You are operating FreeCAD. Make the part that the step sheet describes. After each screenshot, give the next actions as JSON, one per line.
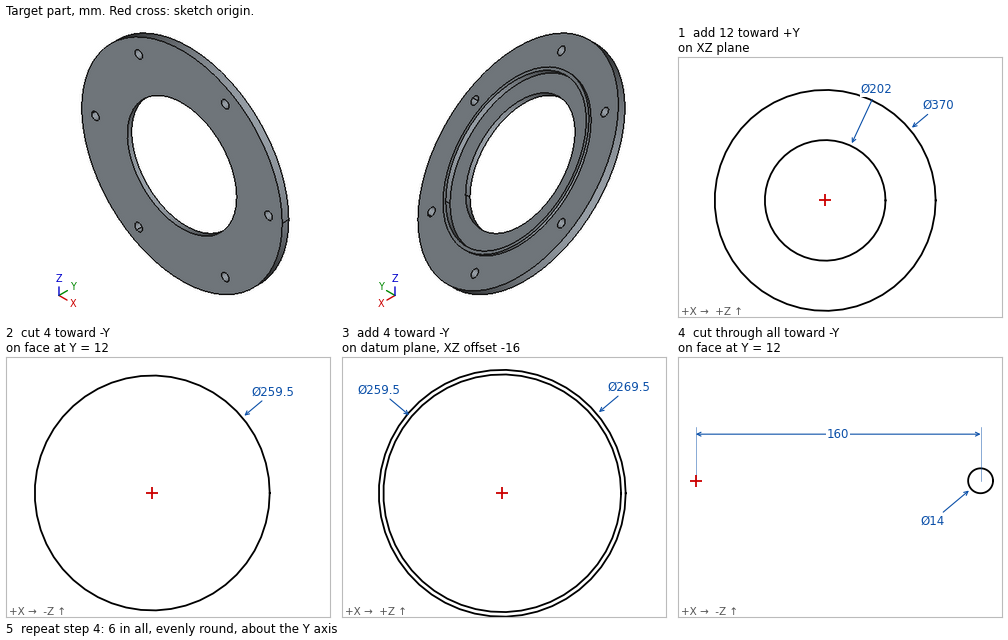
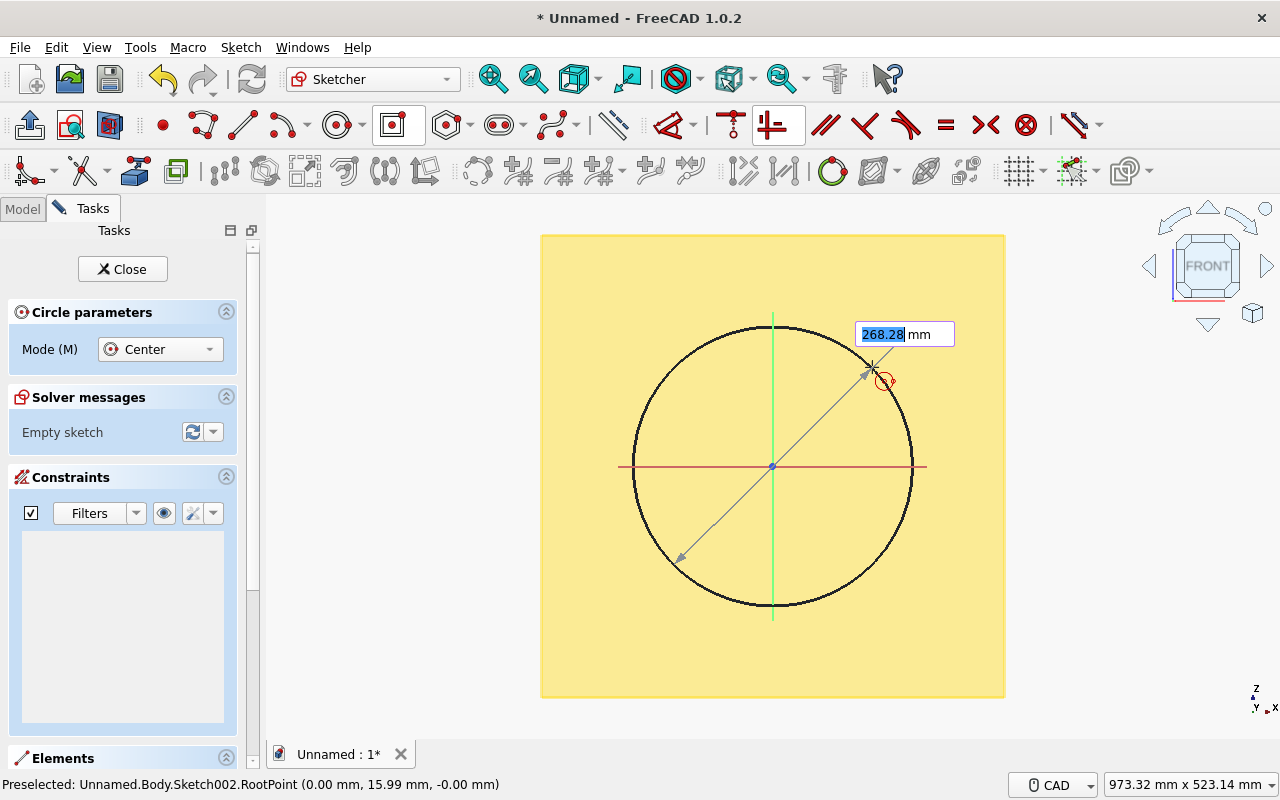
{"action": "type", "text": "269.5"}
{"action": "key", "text": "Return"}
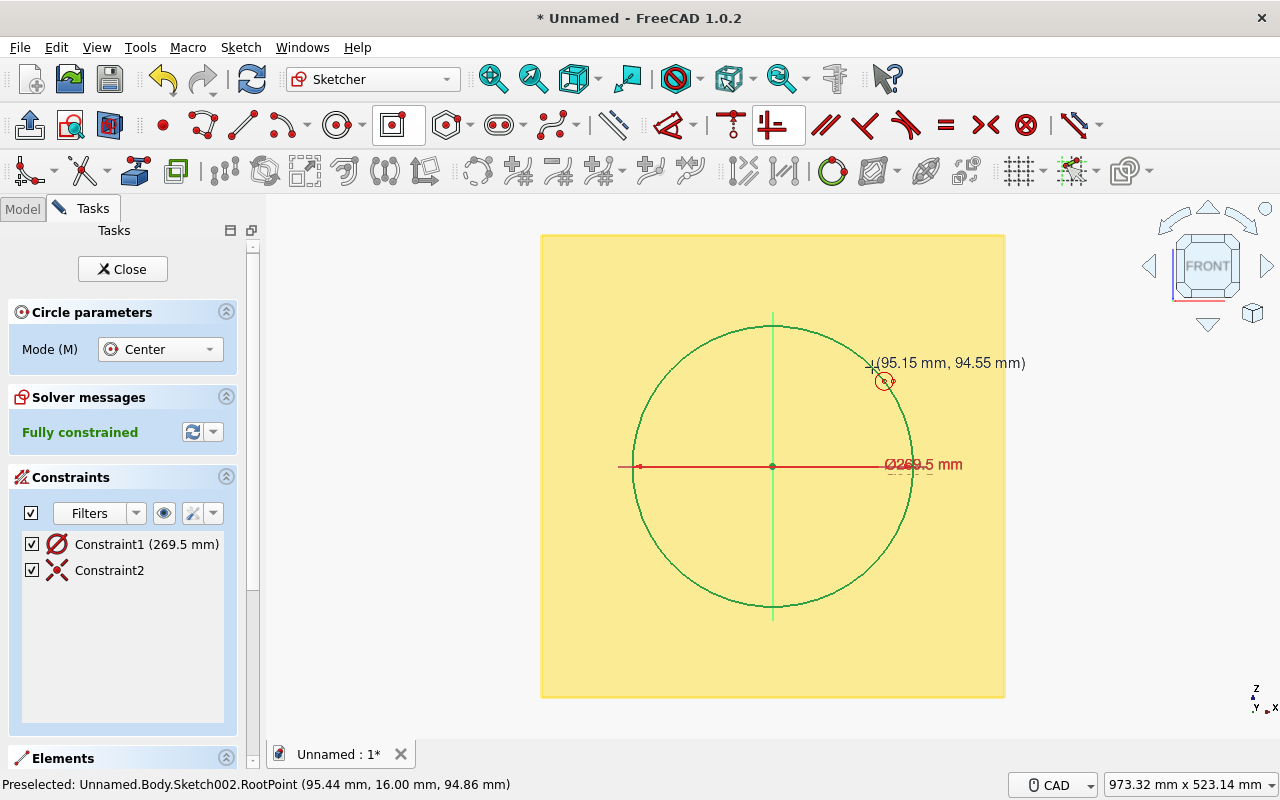
{"action": "left_click", "coordinate": [773, 467]}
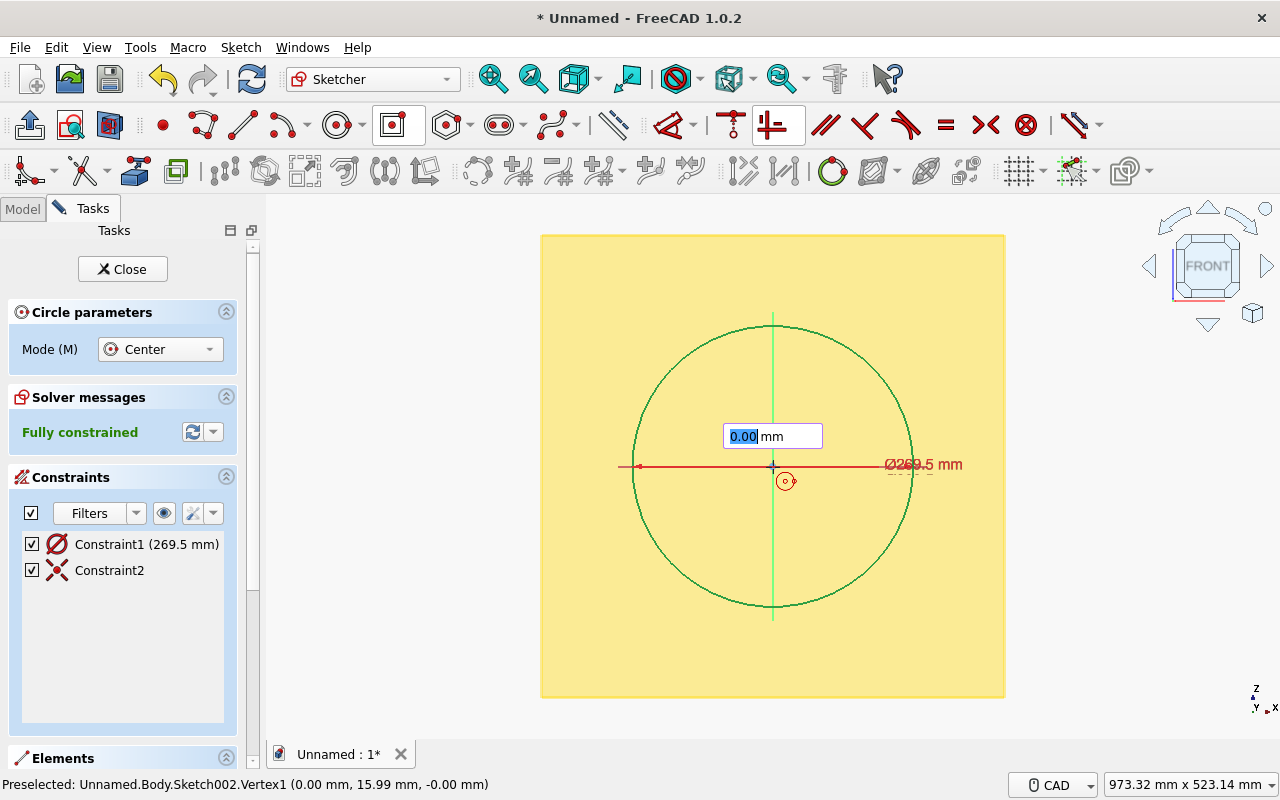
{"action": "scroll", "coordinate": [868, 371], "scroll_direction": "up", "scroll_amount": 6}
{"action": "mouse_move", "coordinate": [868, 370]}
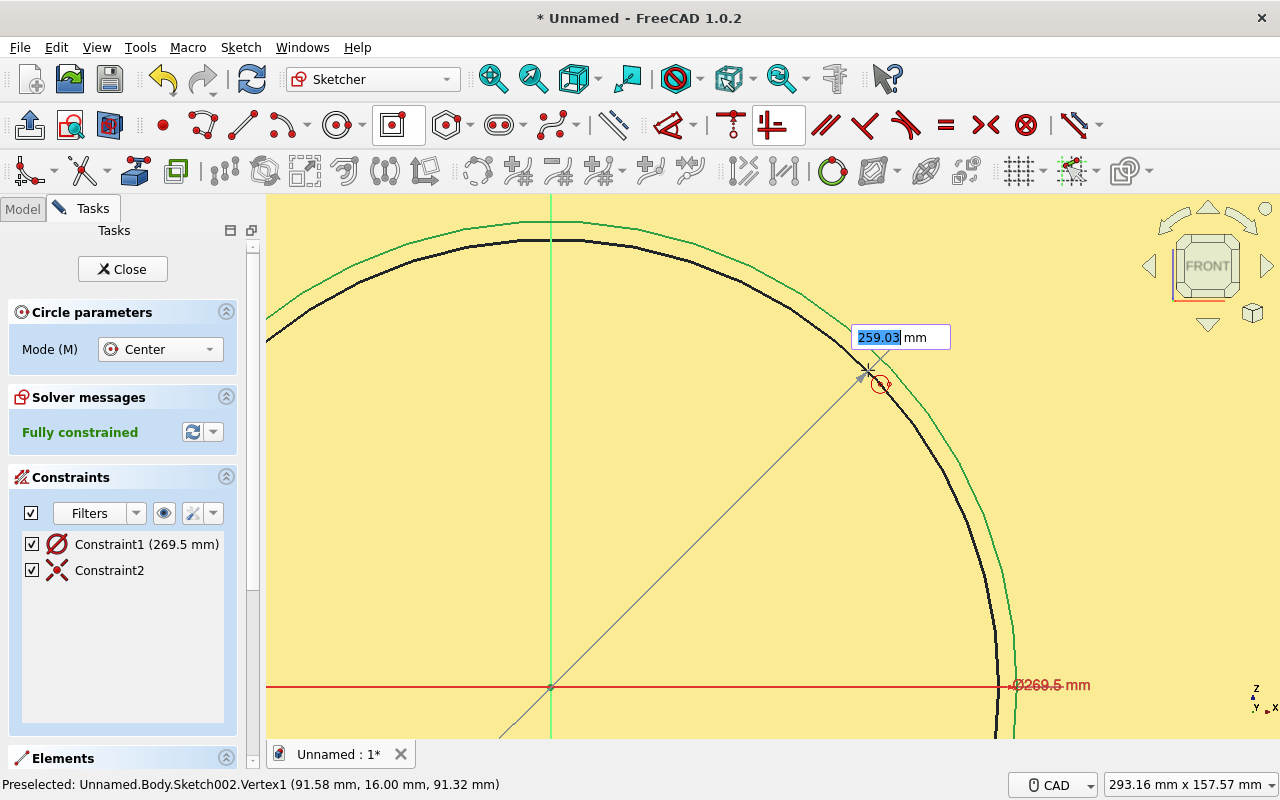
{"action": "type", "text": "259.5"}
{"action": "key", "text": "Return"}
{"action": "key", "text": "Escape"}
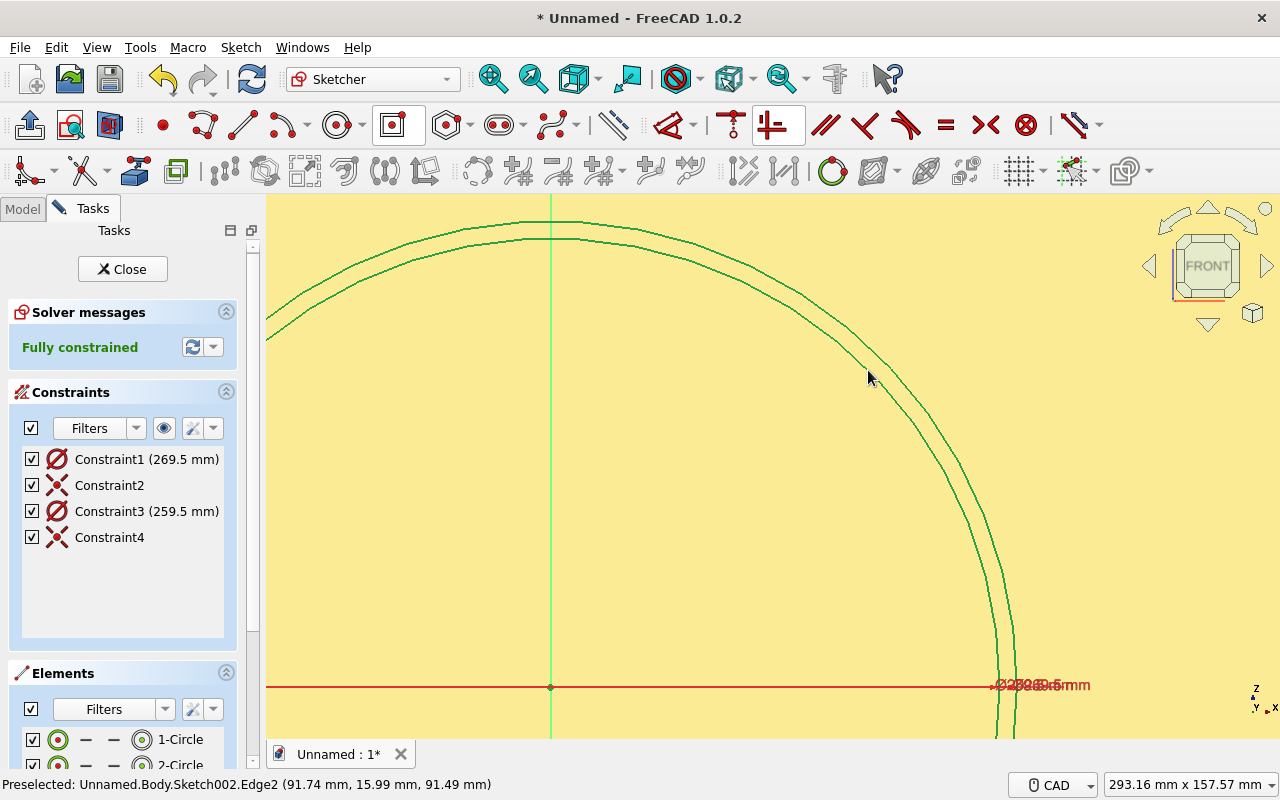
{"action": "left_click", "coordinate": [123, 269]}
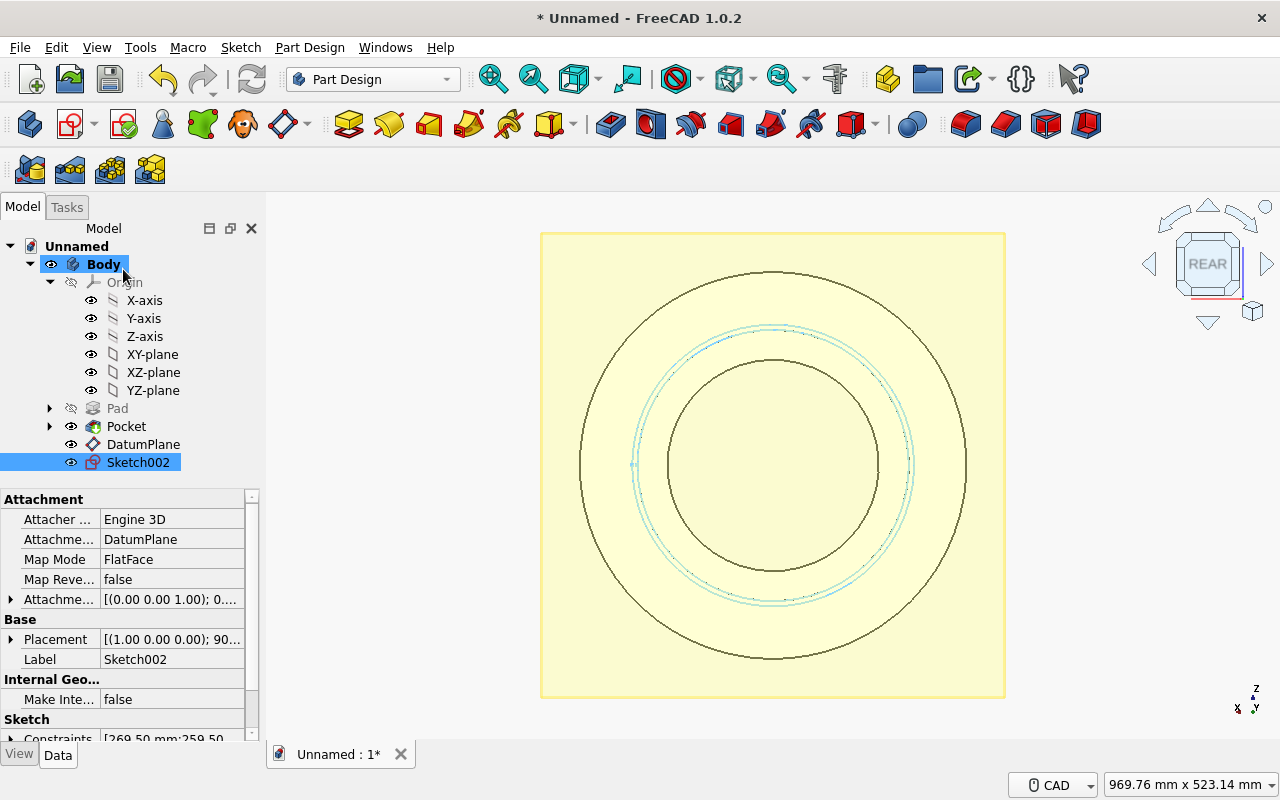
{"action": "left_click", "coordinate": [350, 124]}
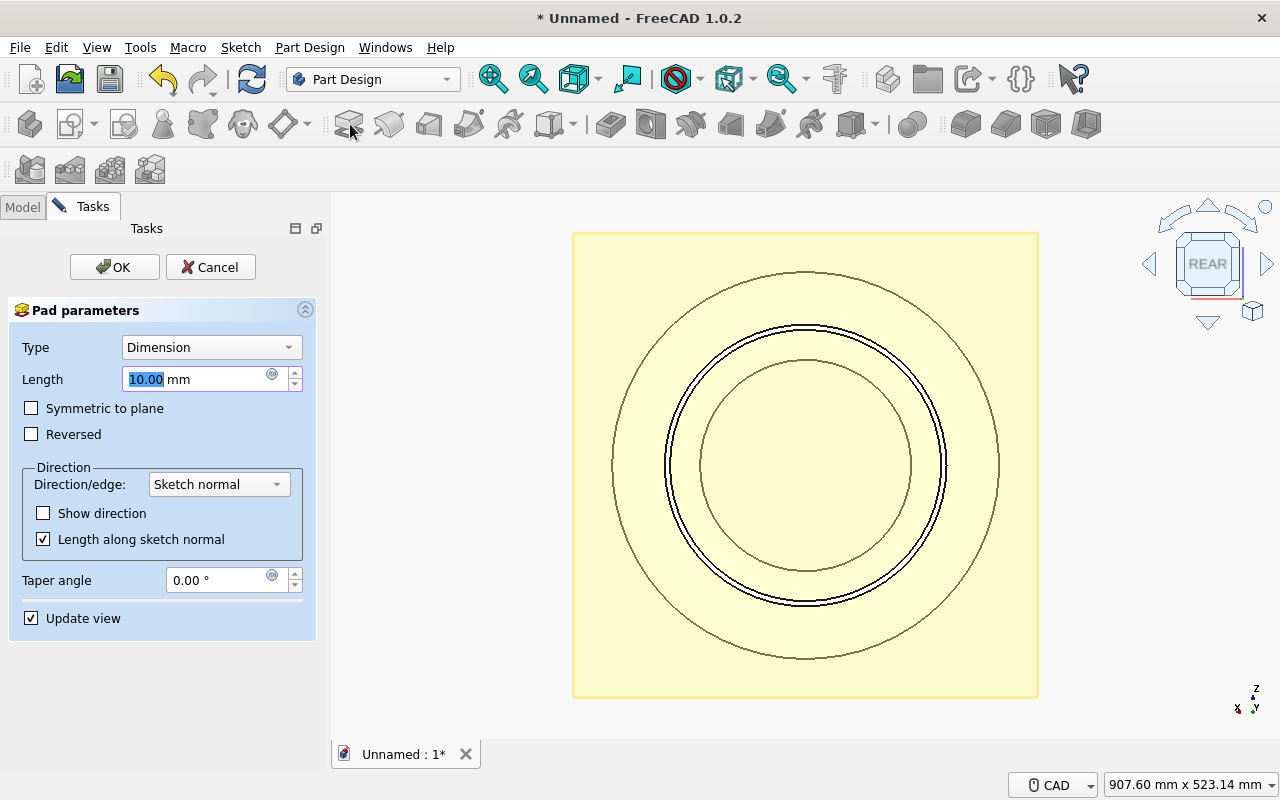
{"action": "type", "text": "4"}
{"action": "key", "text": "Tab"}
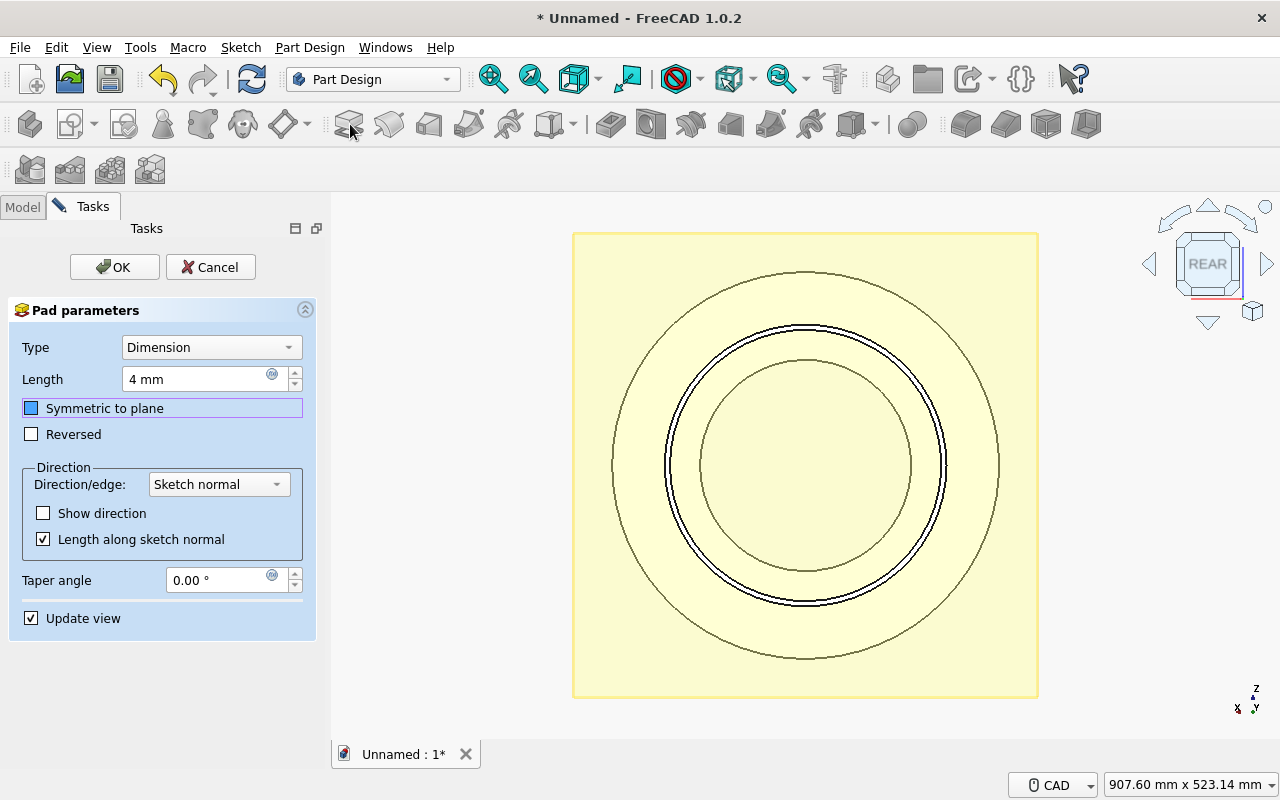
{"action": "left_click", "coordinate": [115, 267]}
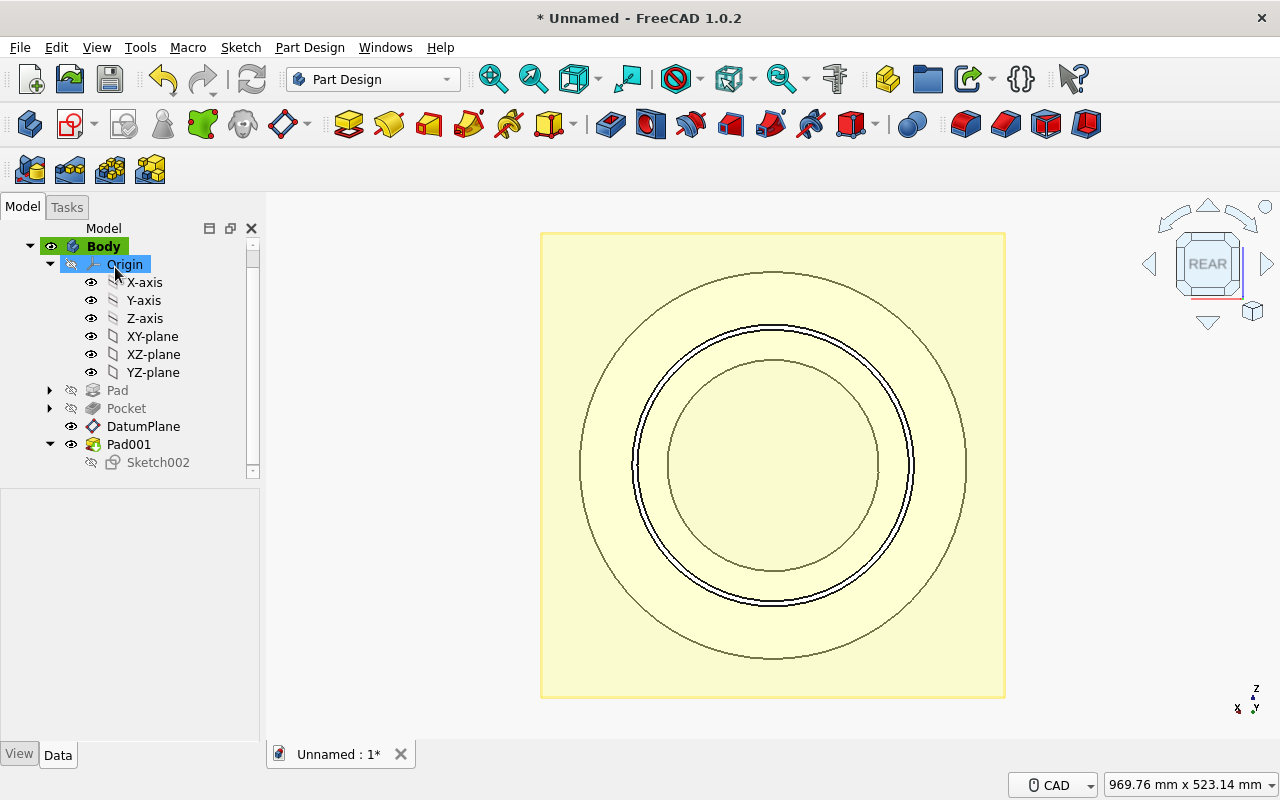
{"action": "left_click", "coordinate": [116, 426]}
{"action": "key", "text": "space"}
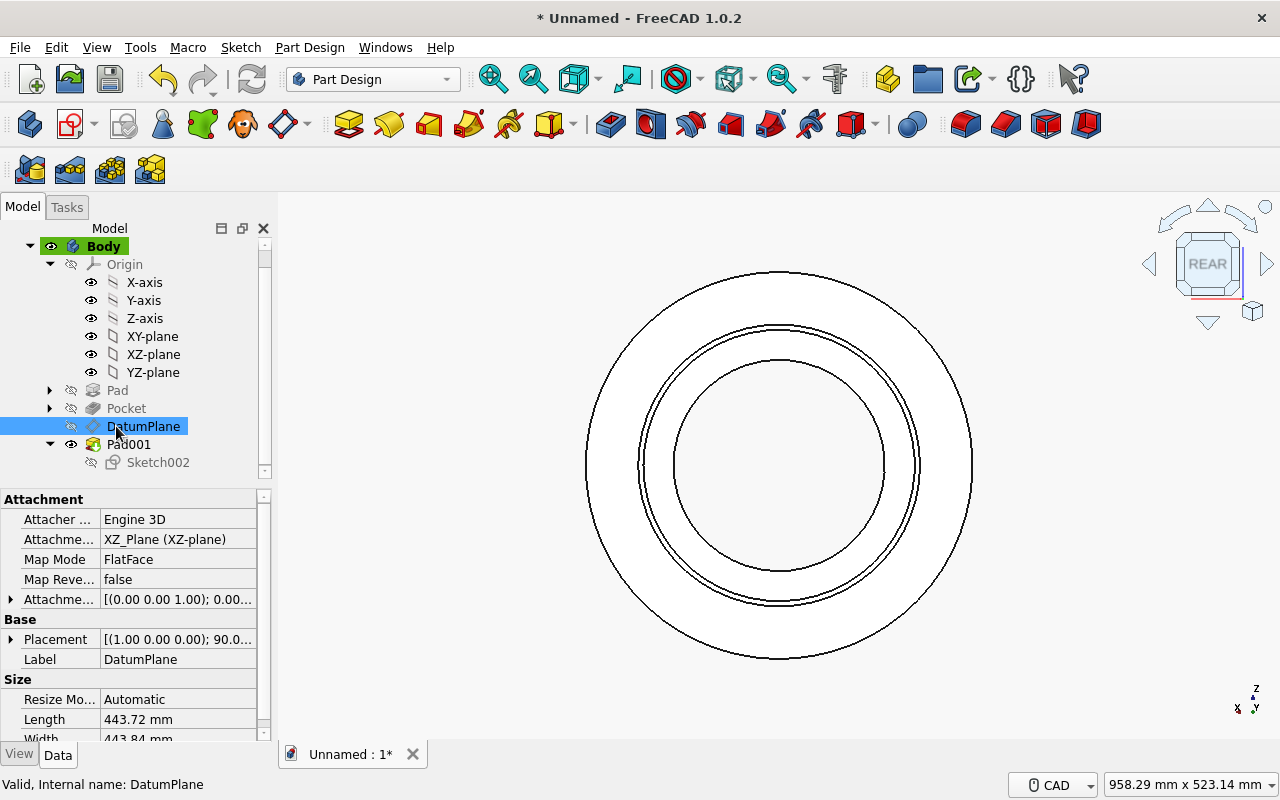
{"action": "left_click", "coordinate": [779, 630]}